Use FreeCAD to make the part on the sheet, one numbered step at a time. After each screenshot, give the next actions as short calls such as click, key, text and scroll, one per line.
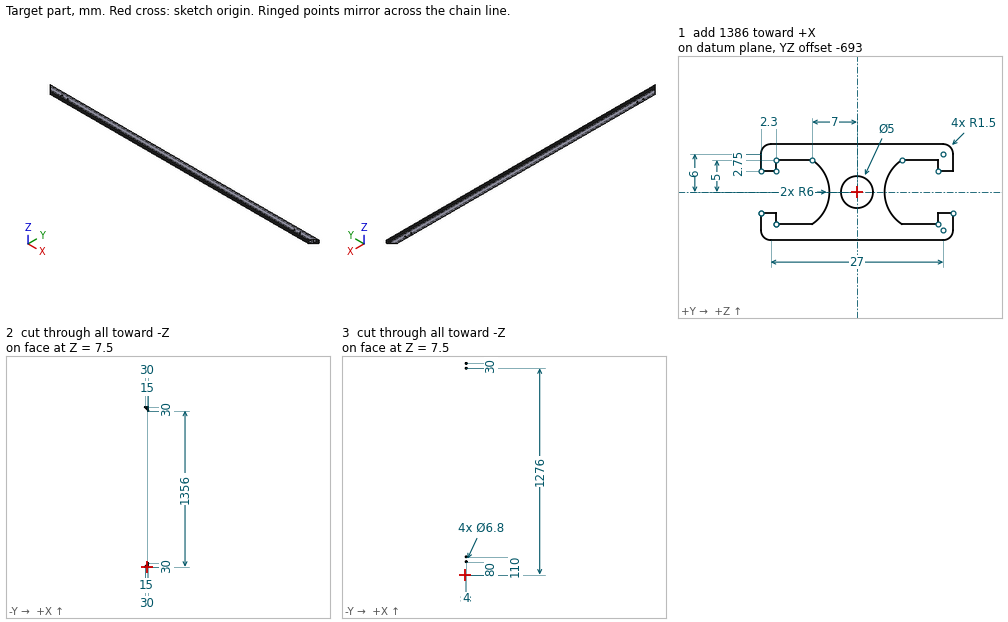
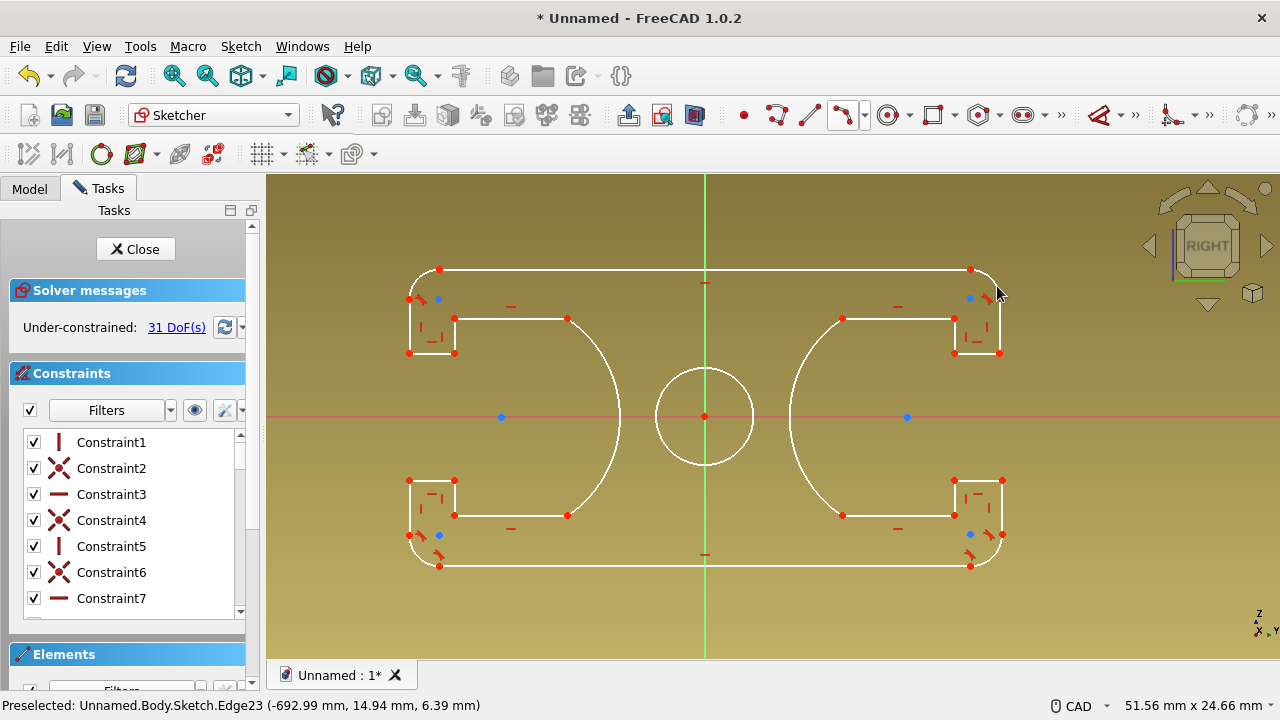
click(811, 270)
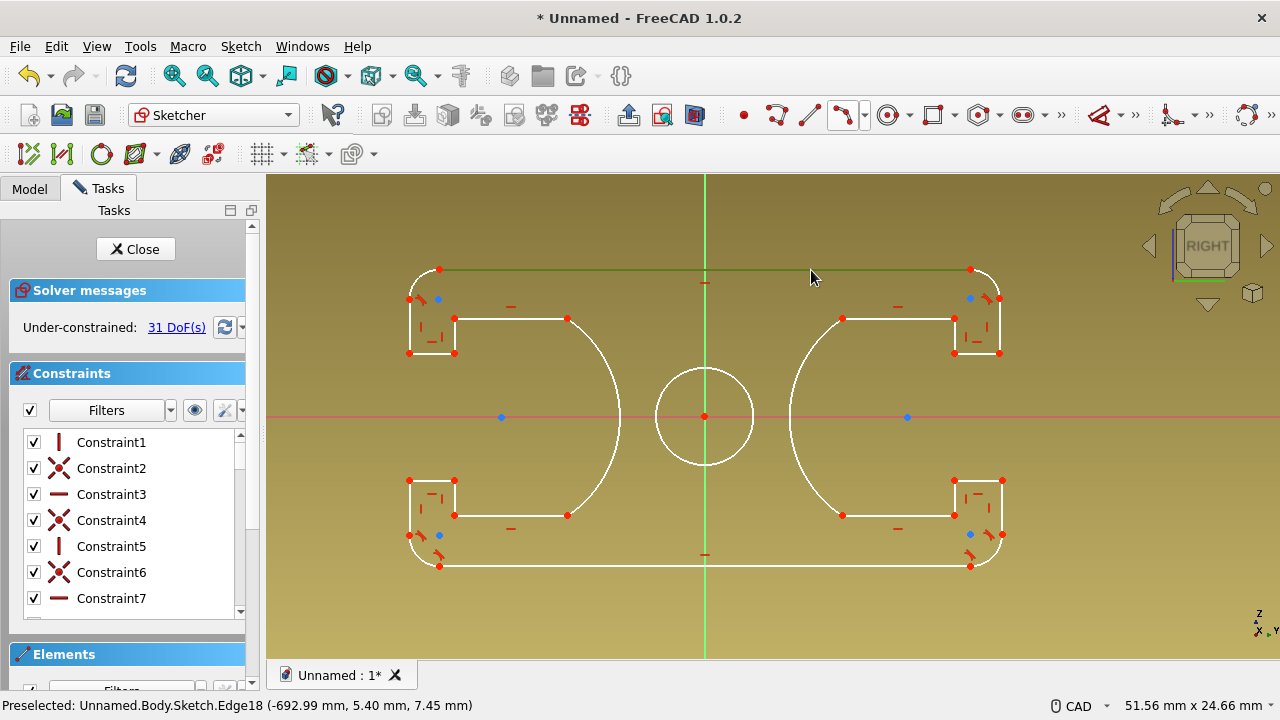
click(996, 286)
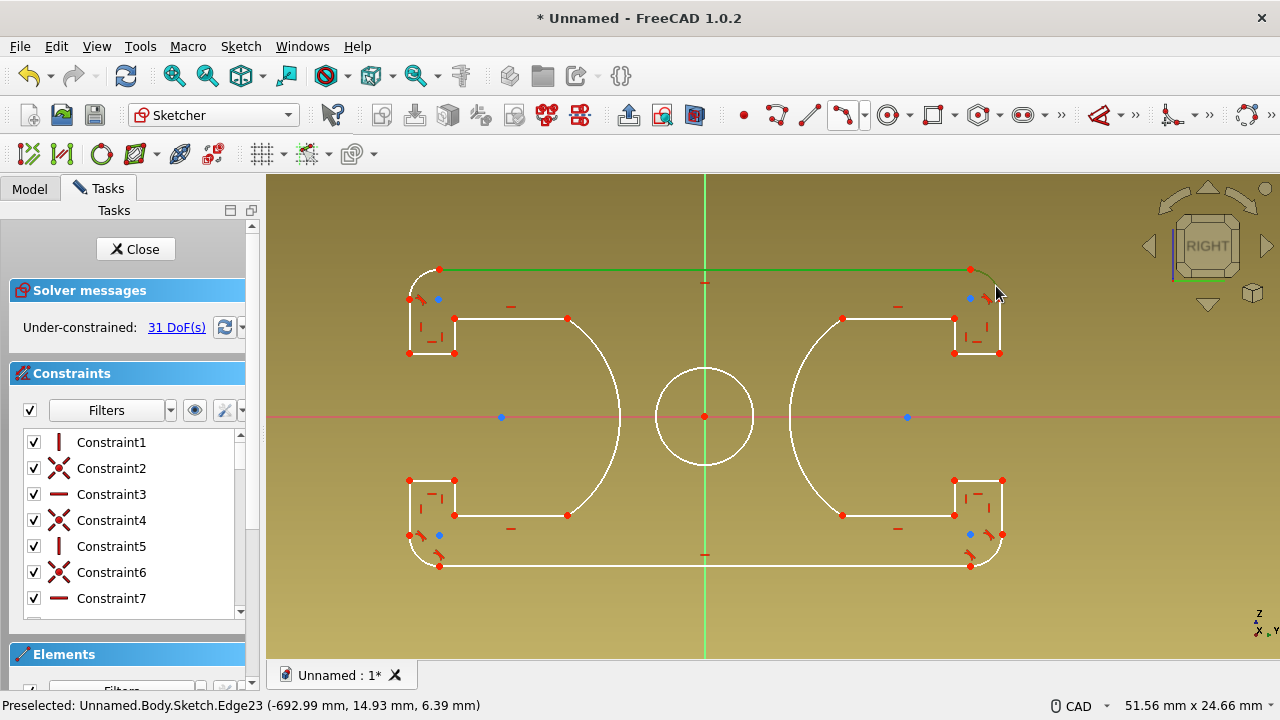
key(t)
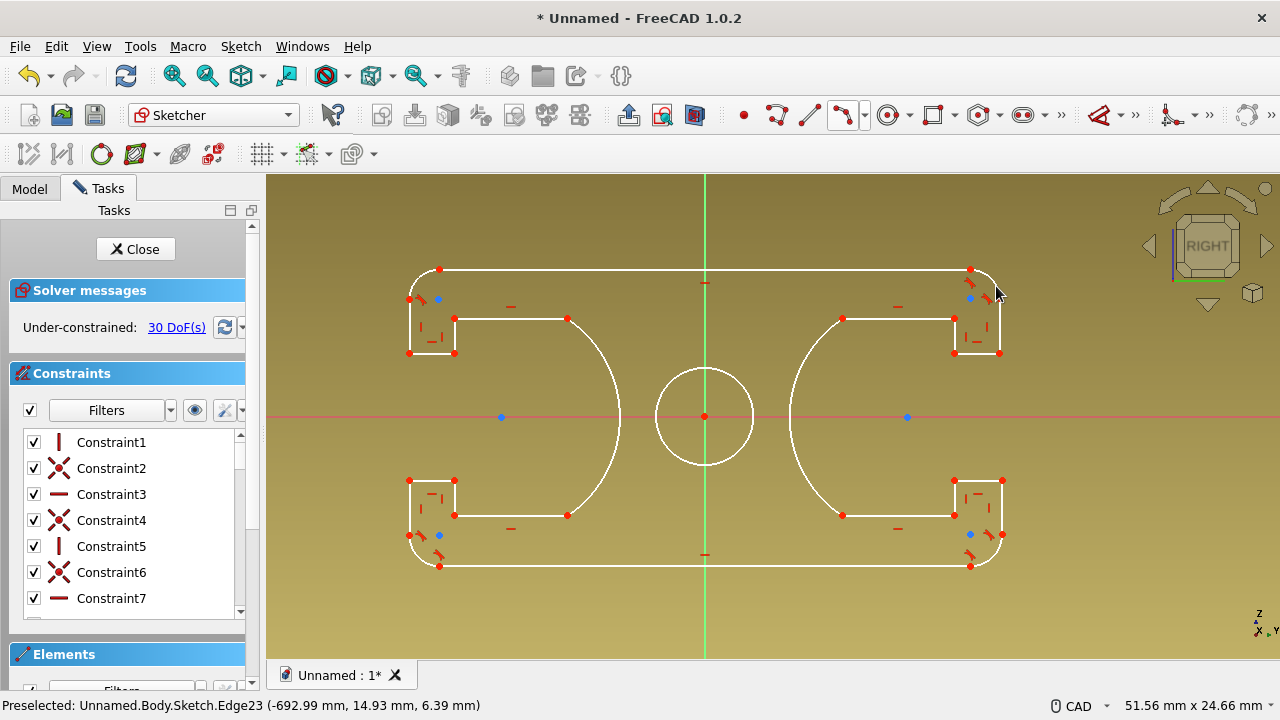
click(811, 270)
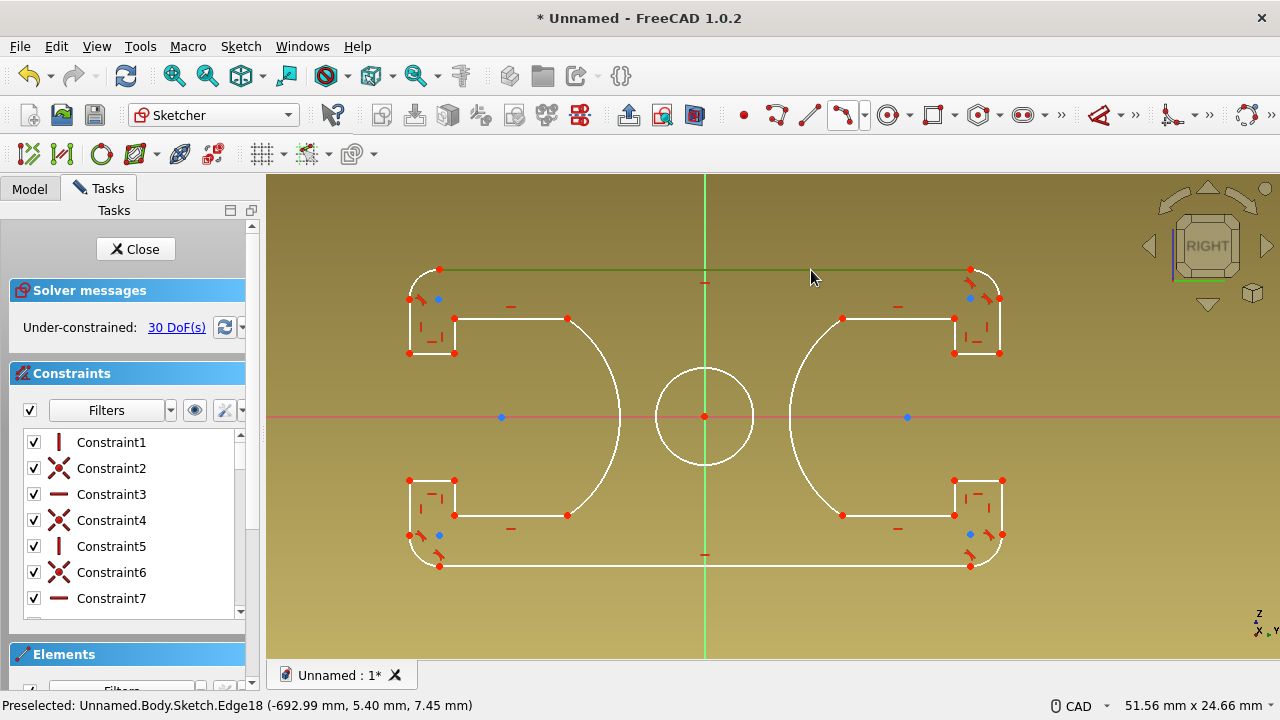
click(426, 273)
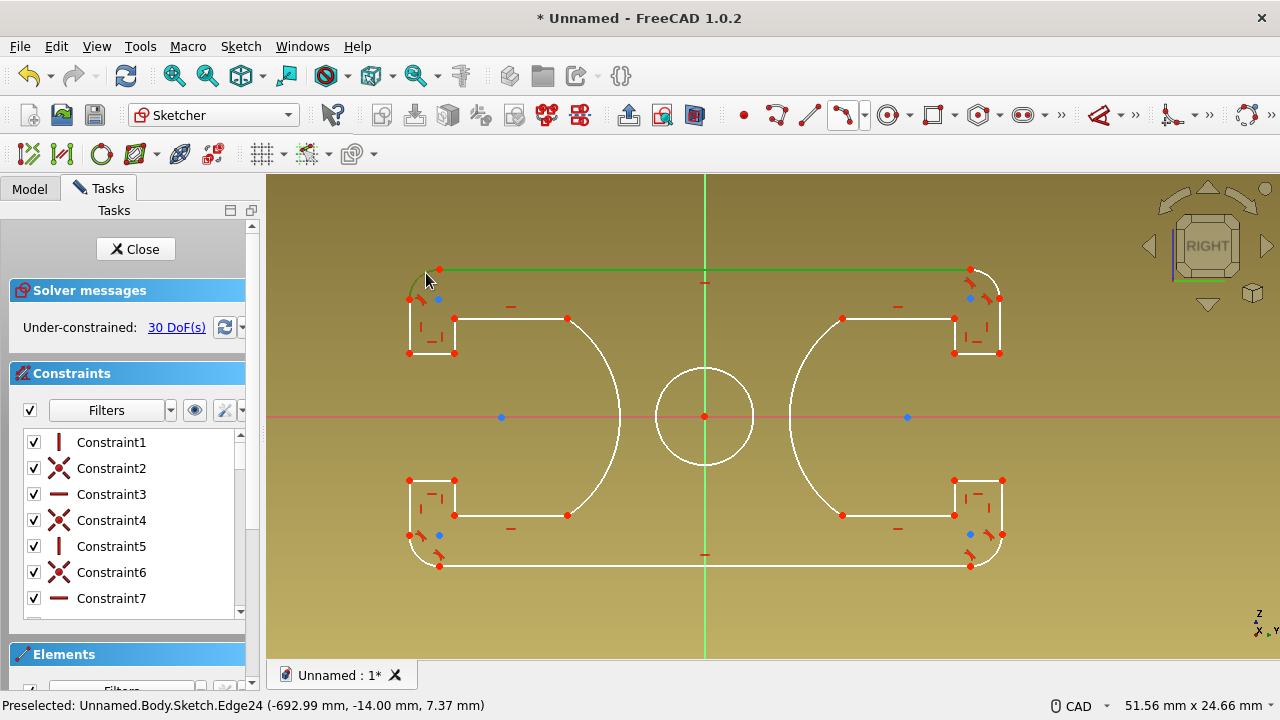
key(t)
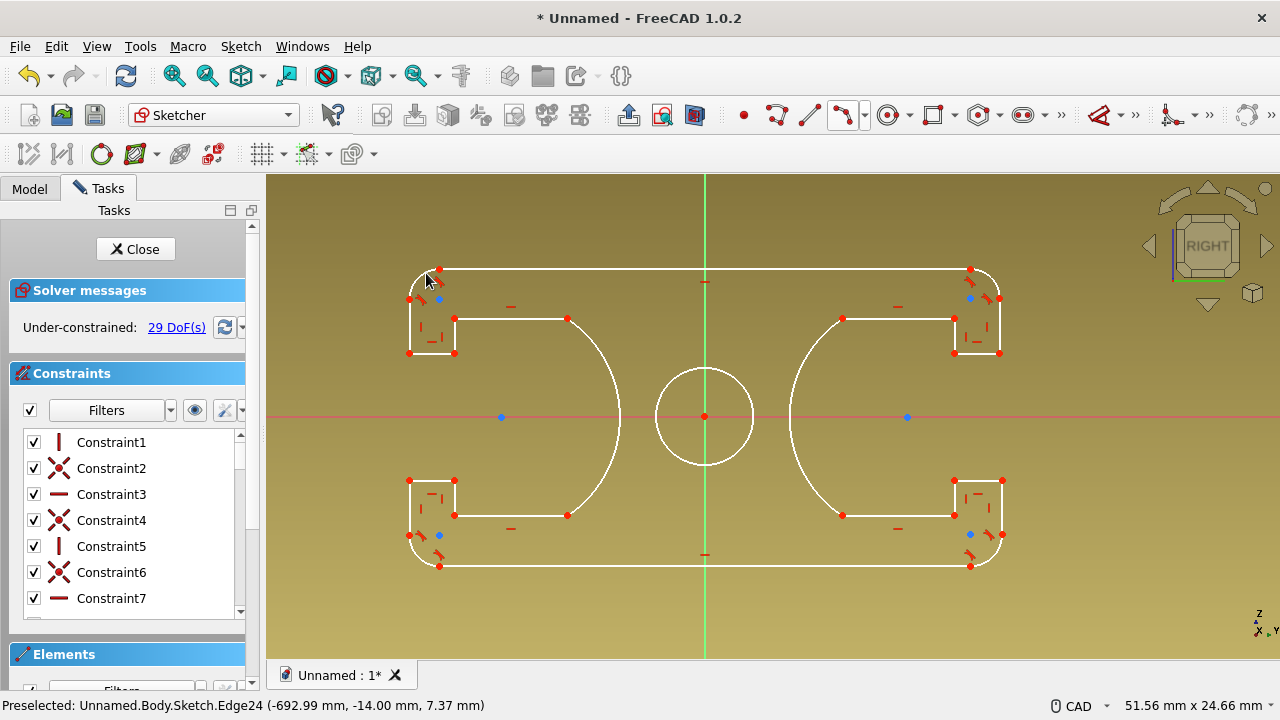
click(413, 550)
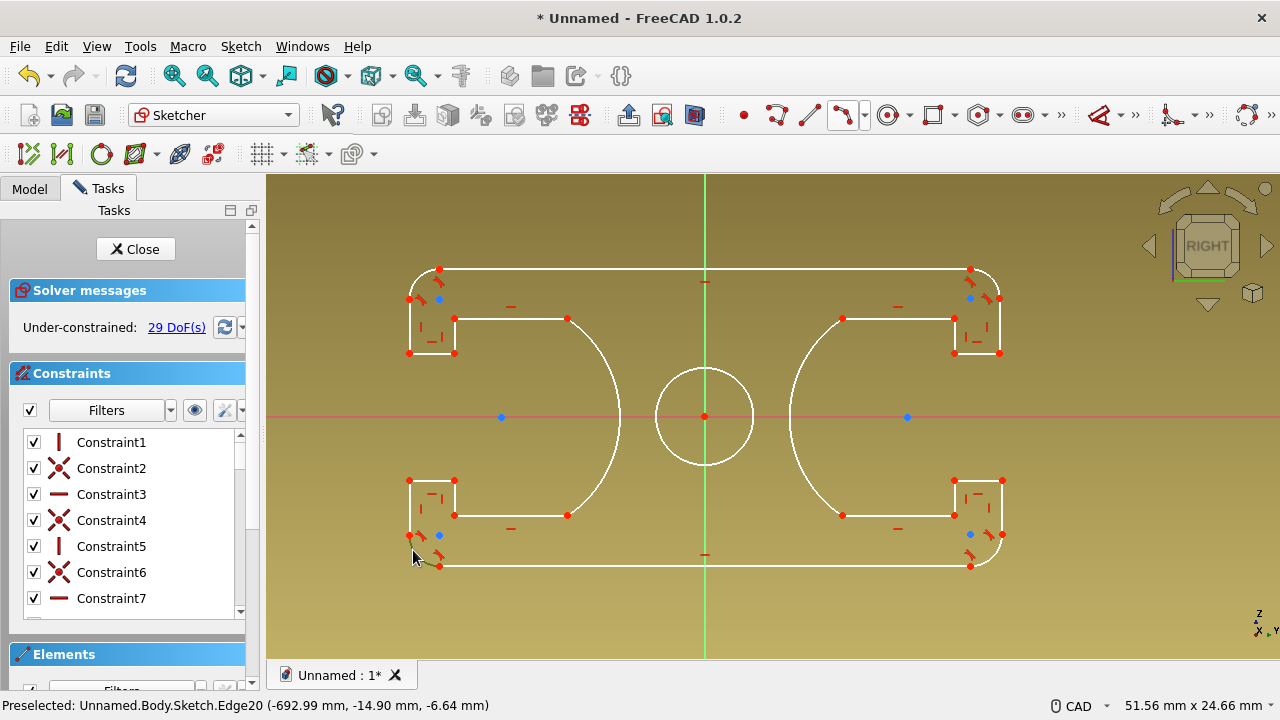
click(985, 563)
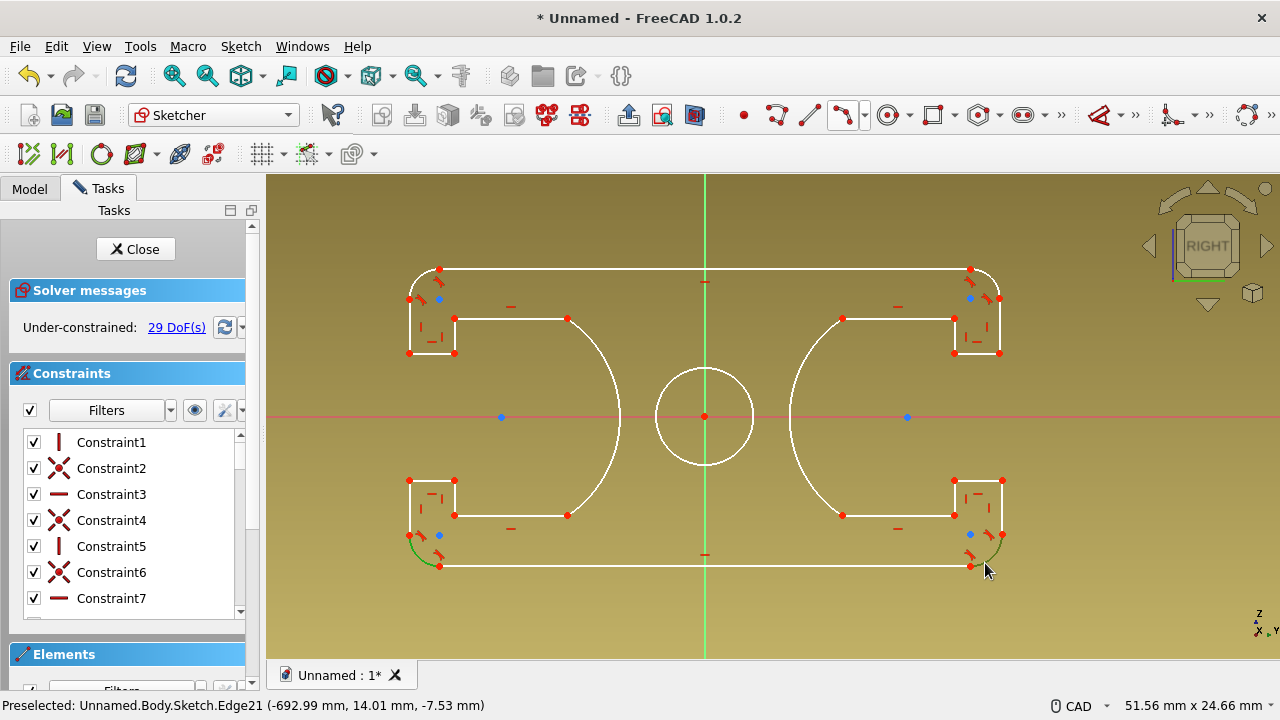
click(996, 285)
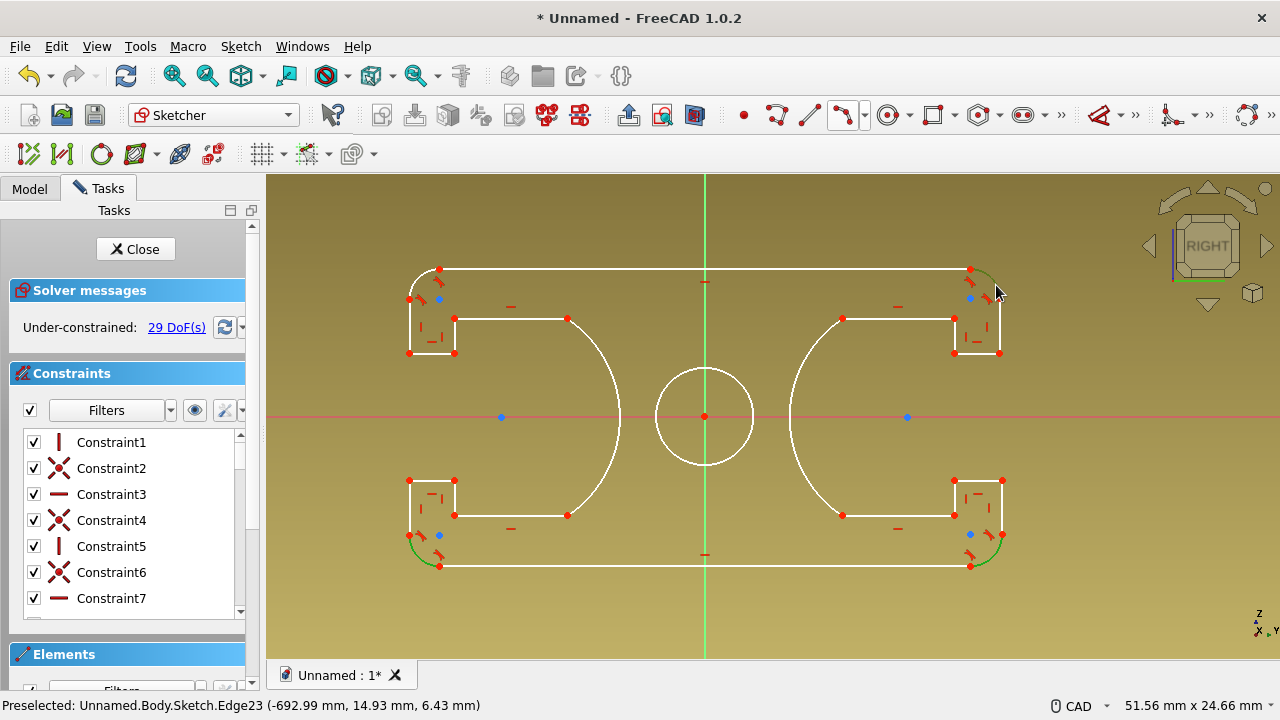
click(426, 272)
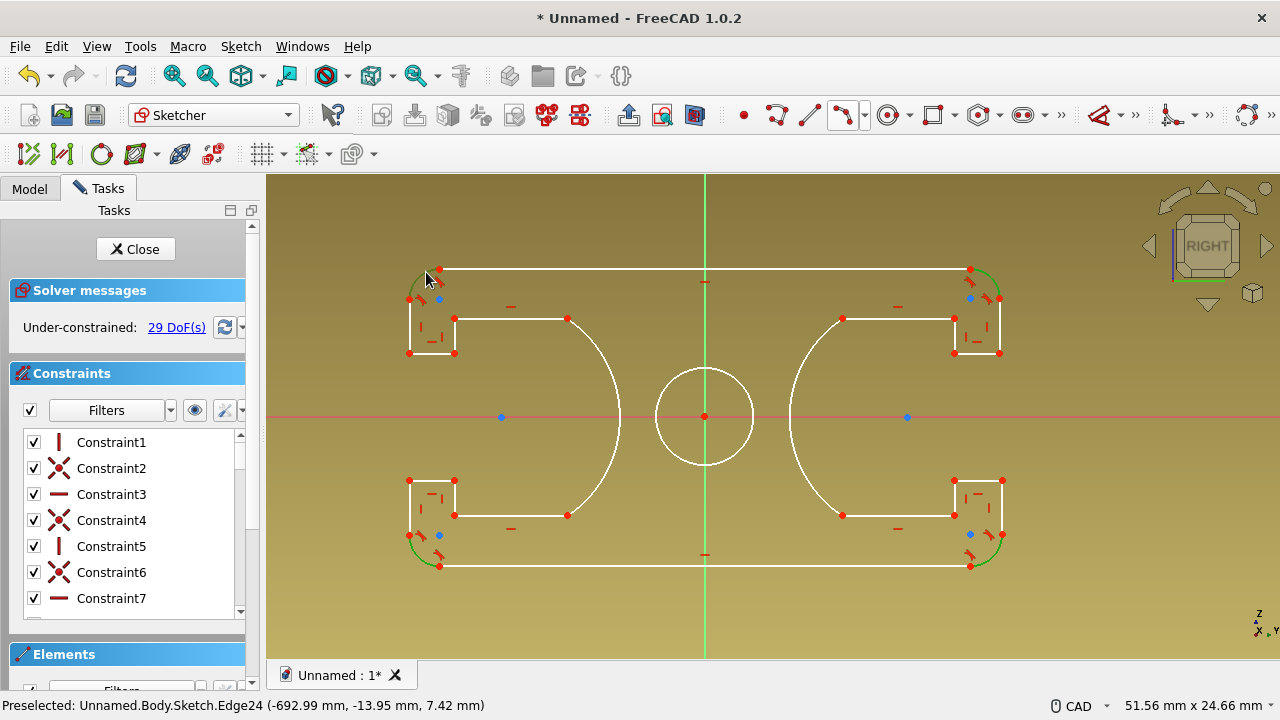
key(e)